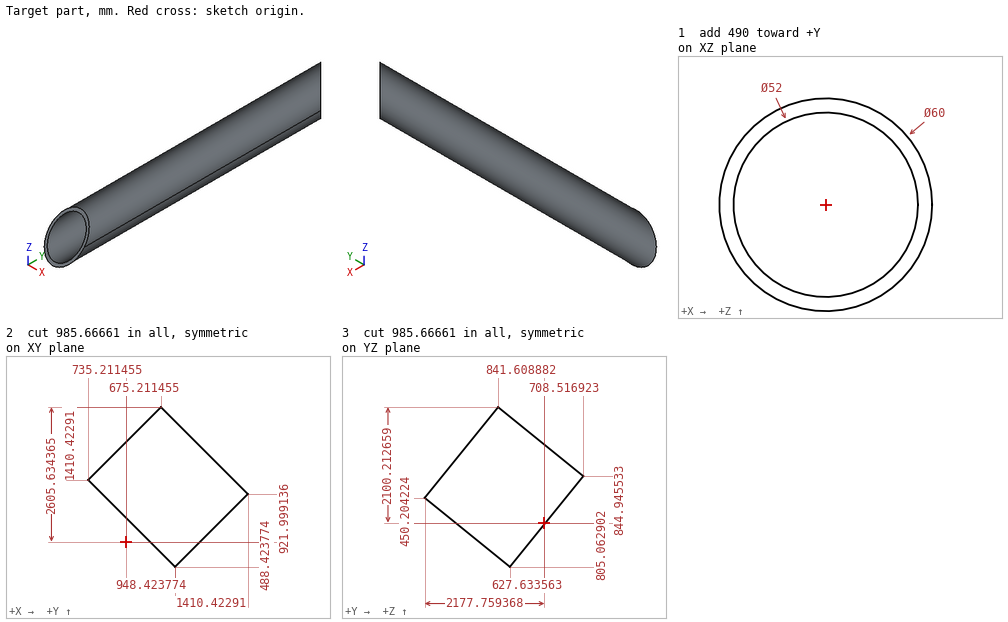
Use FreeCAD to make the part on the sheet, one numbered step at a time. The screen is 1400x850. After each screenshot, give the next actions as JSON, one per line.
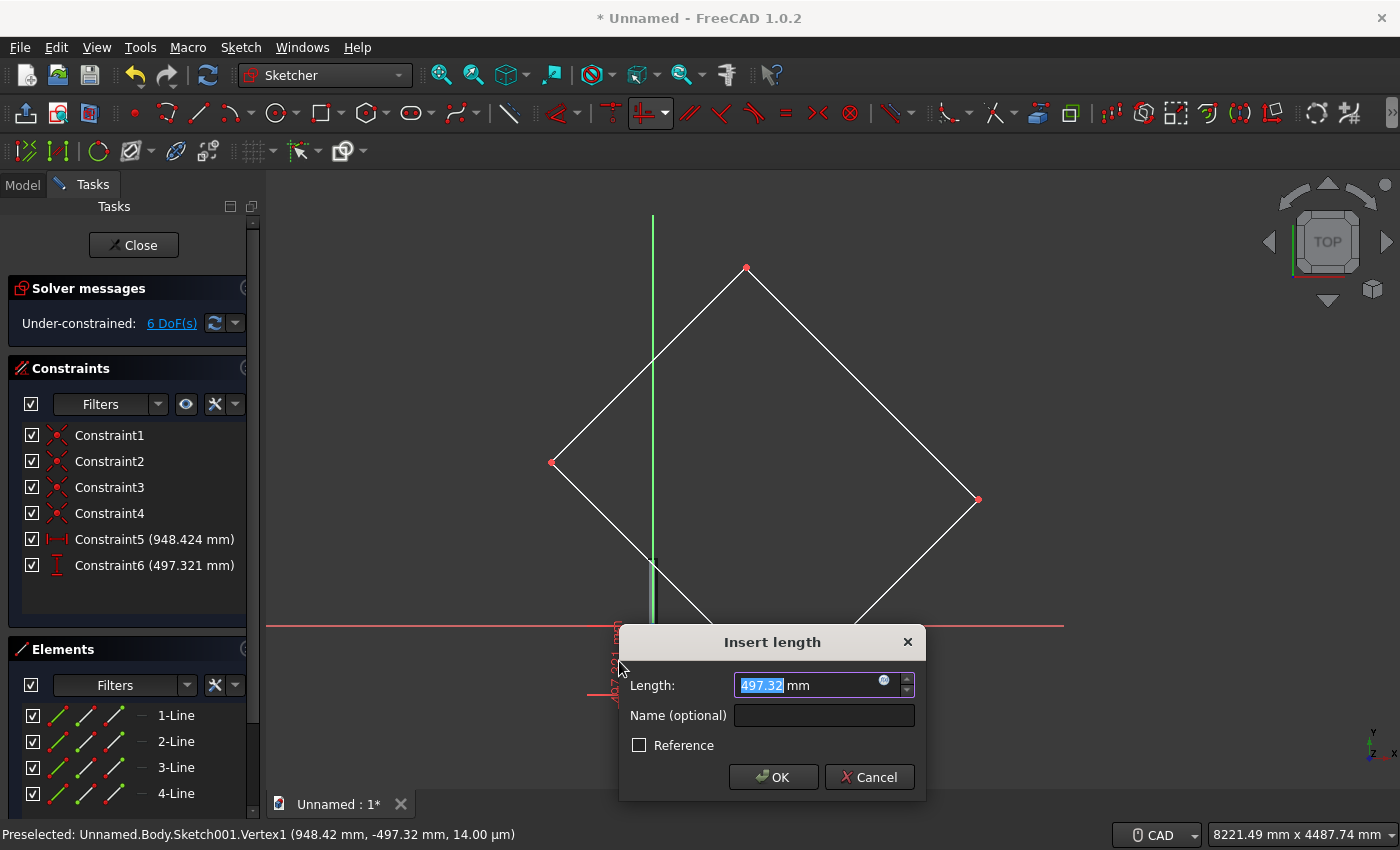
{"action": "type", "text": "488.423774"}
{"action": "key", "text": "Return"}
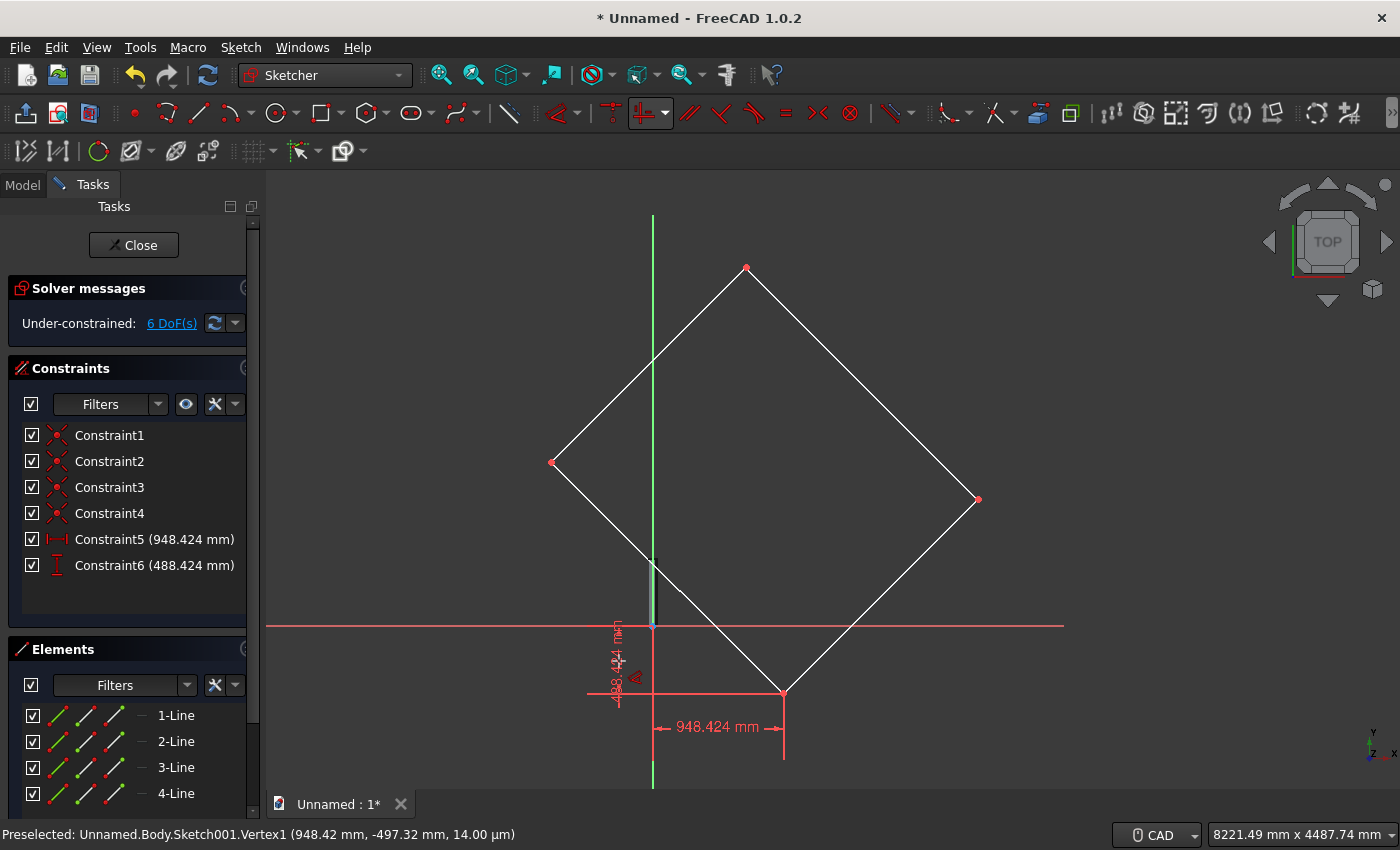
{"action": "left_click", "coordinate": [978, 500]}
{"action": "left_click", "coordinate": [1012, 563]}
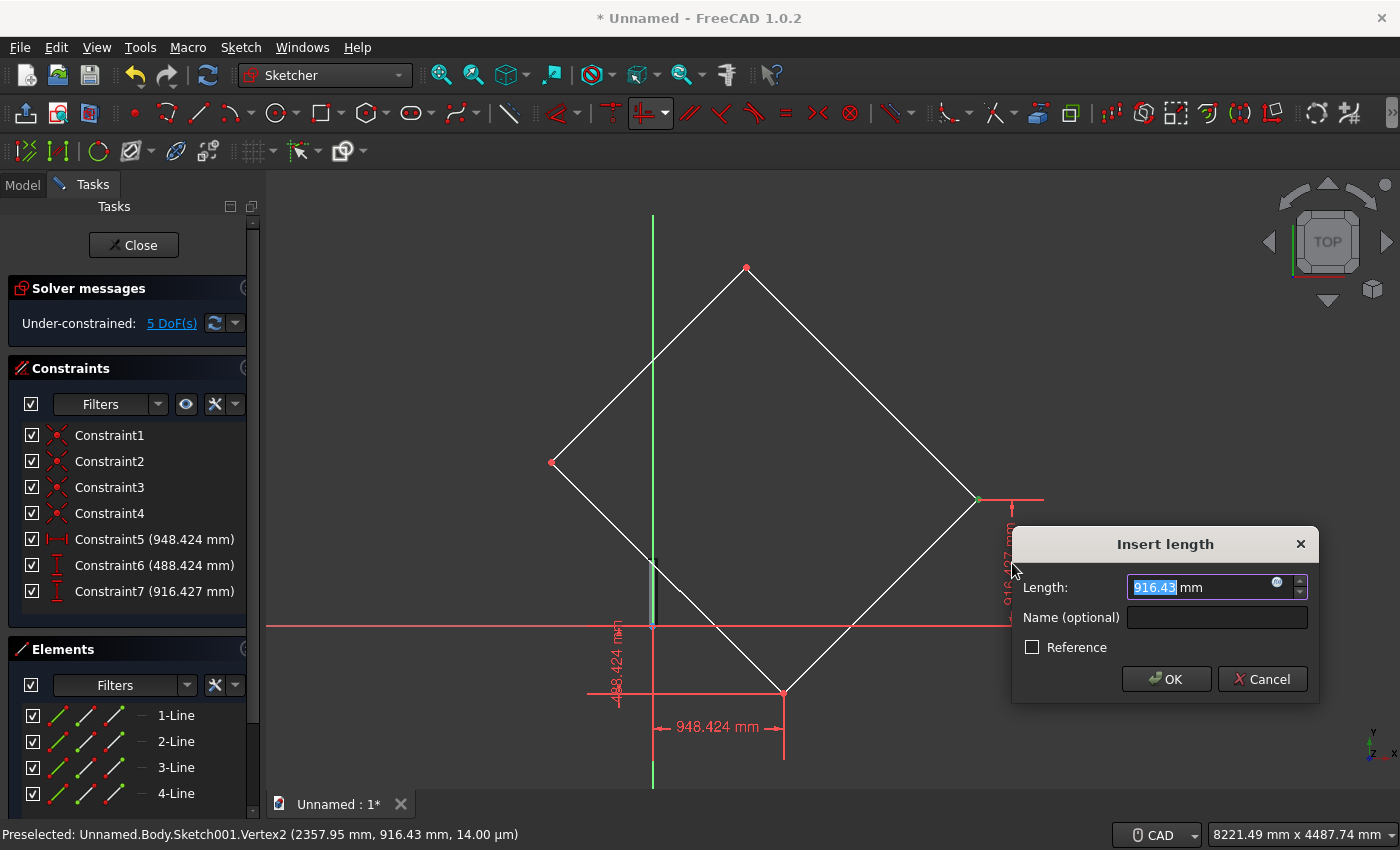
{"action": "type", "text": "921.999136"}
{"action": "key", "text": "Return"}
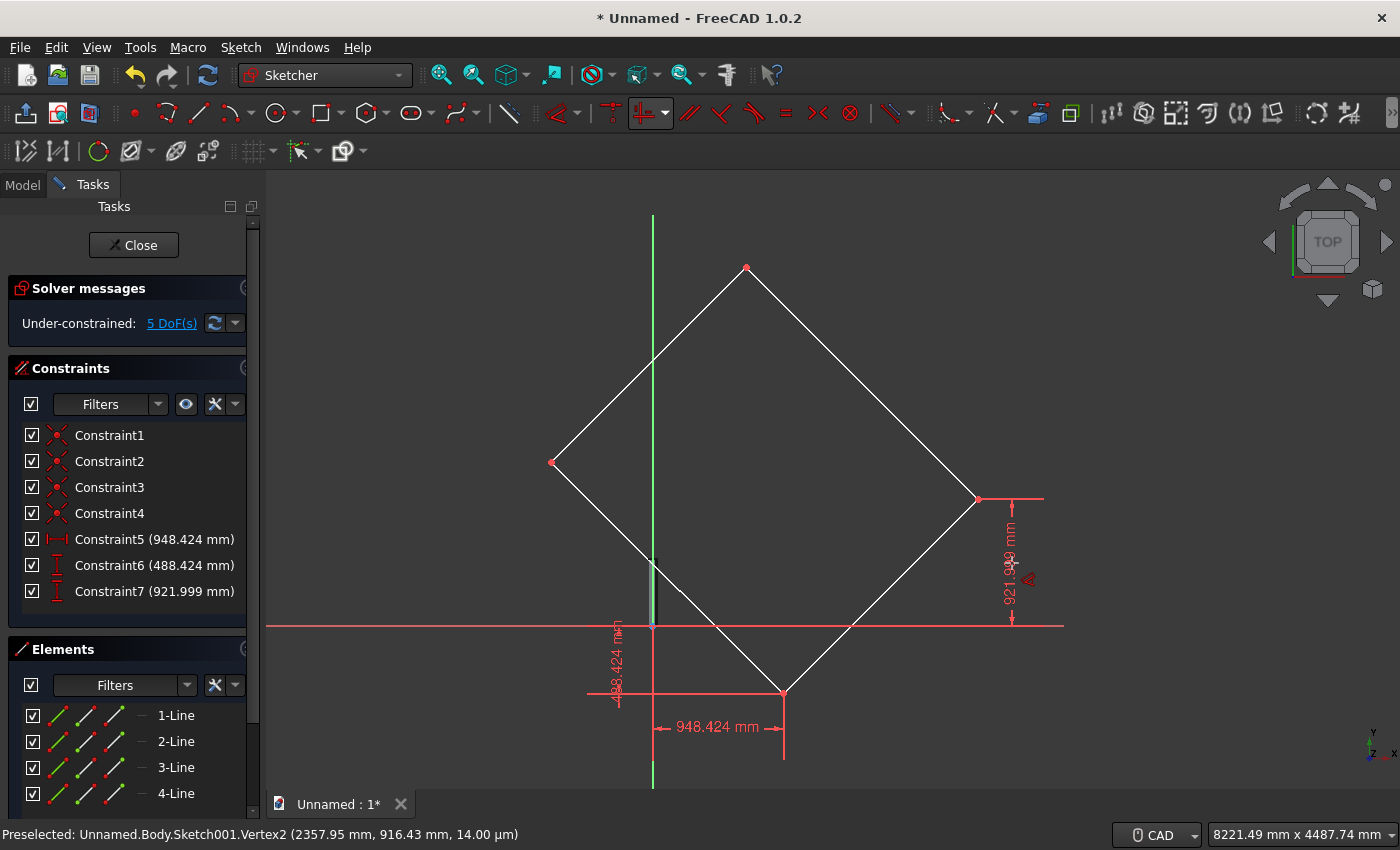
{"action": "left_click", "coordinate": [746, 268]}
{"action": "left_click", "coordinate": [699, 234]}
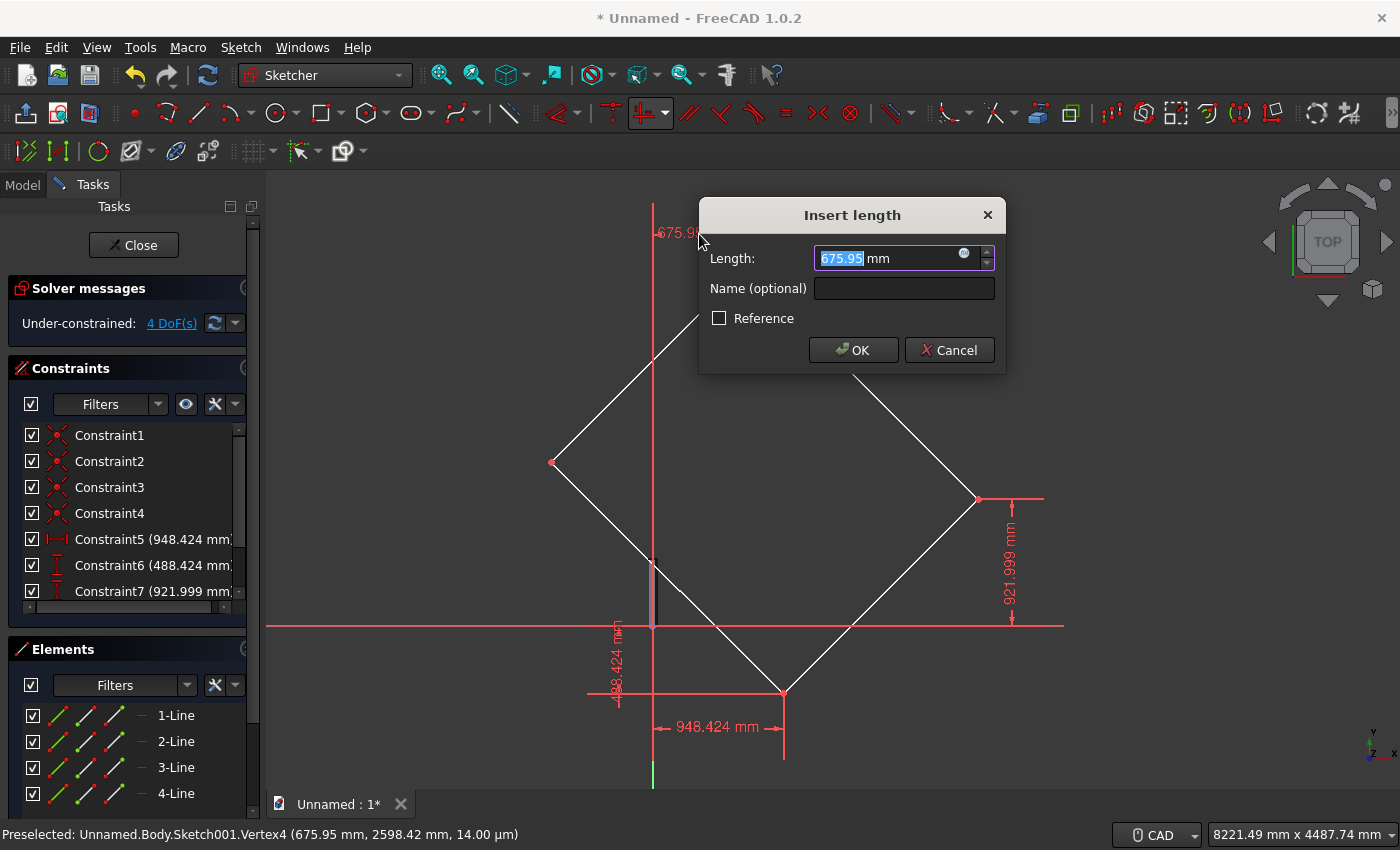
{"action": "type", "text": "675.211455"}
{"action": "key", "text": "Return"}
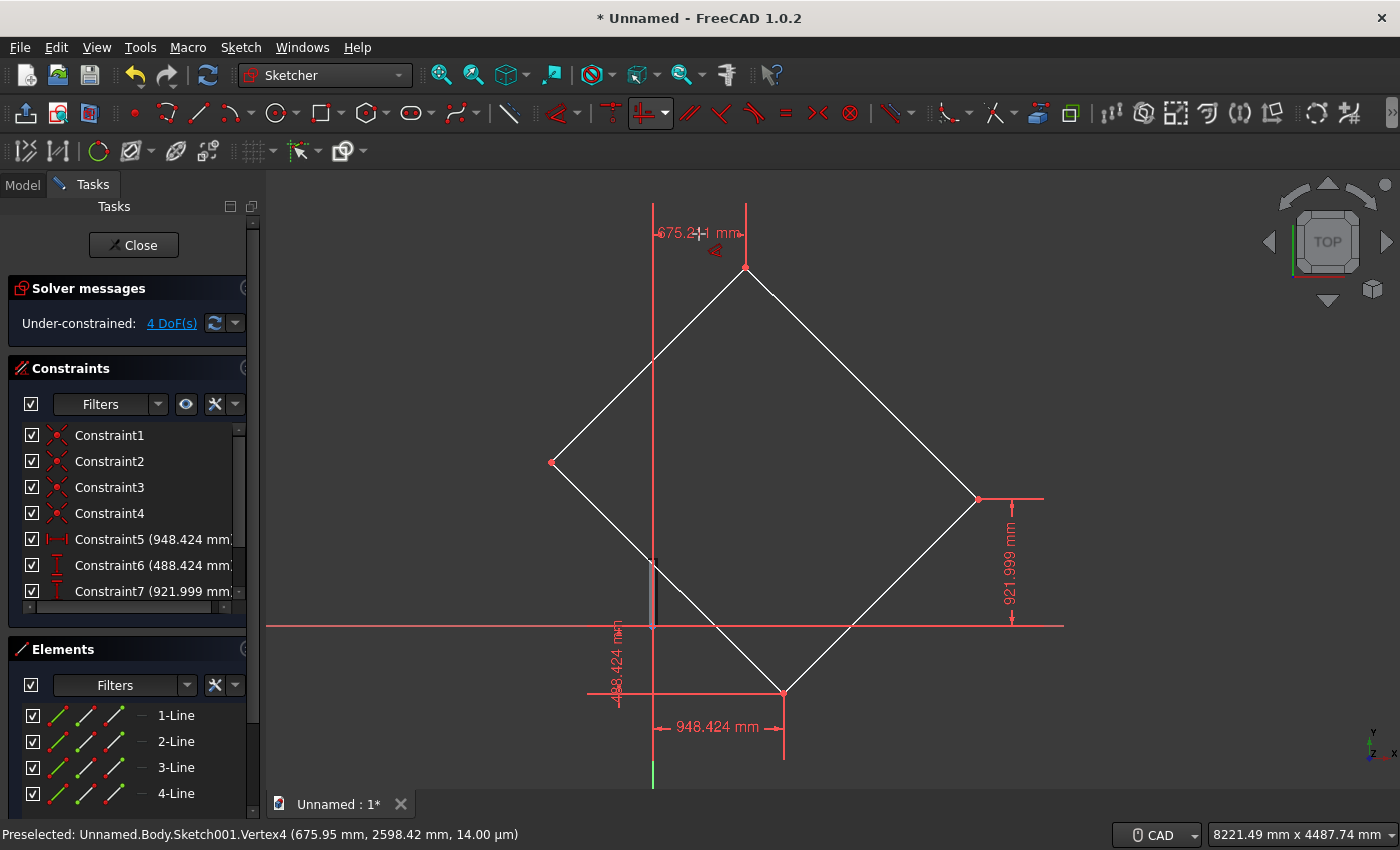
{"action": "left_click", "coordinate": [551, 463]}
{"action": "left_click", "coordinate": [625, 429]}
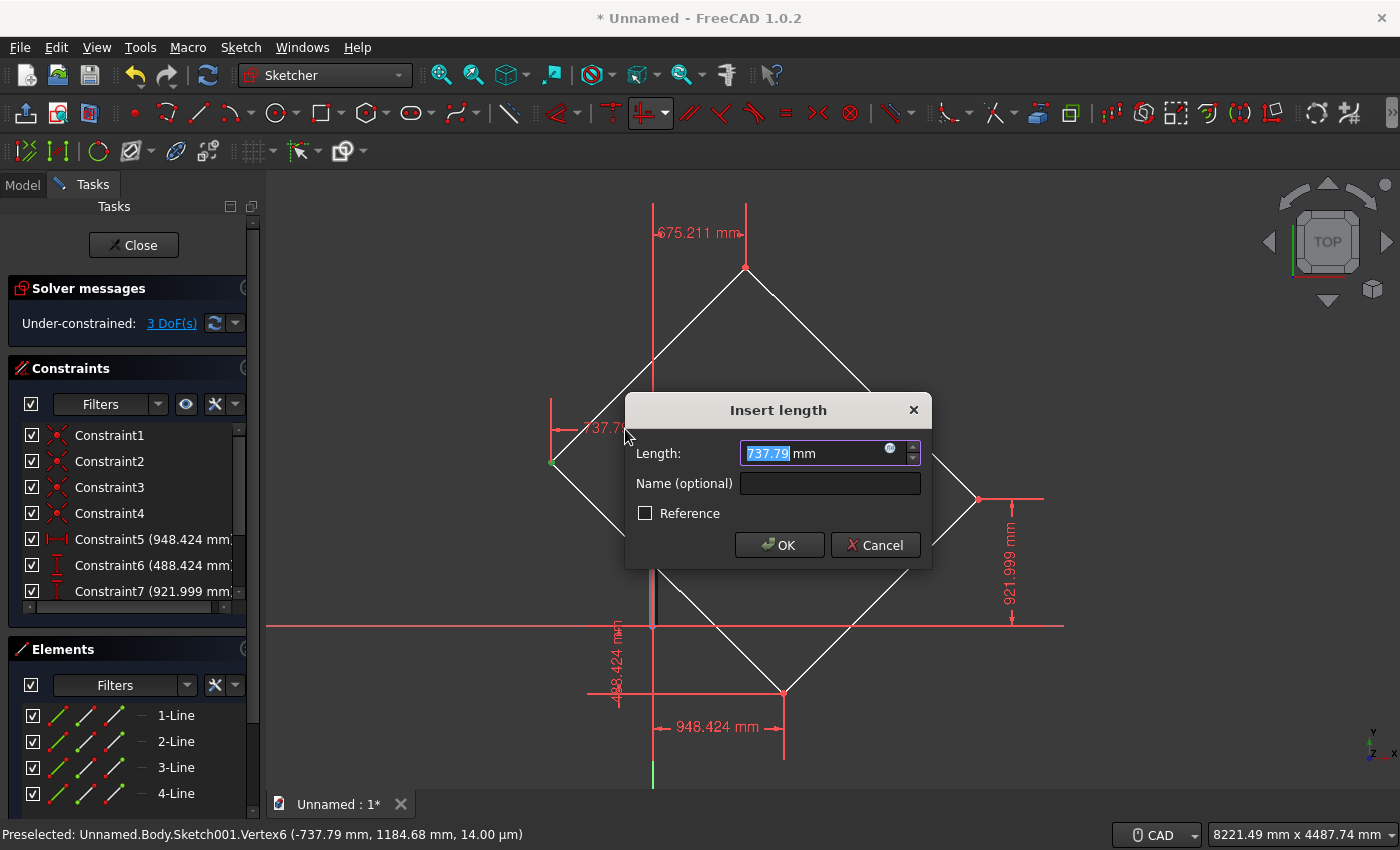
{"action": "type", "text": "735.211455"}
{"action": "key", "text": "Return"}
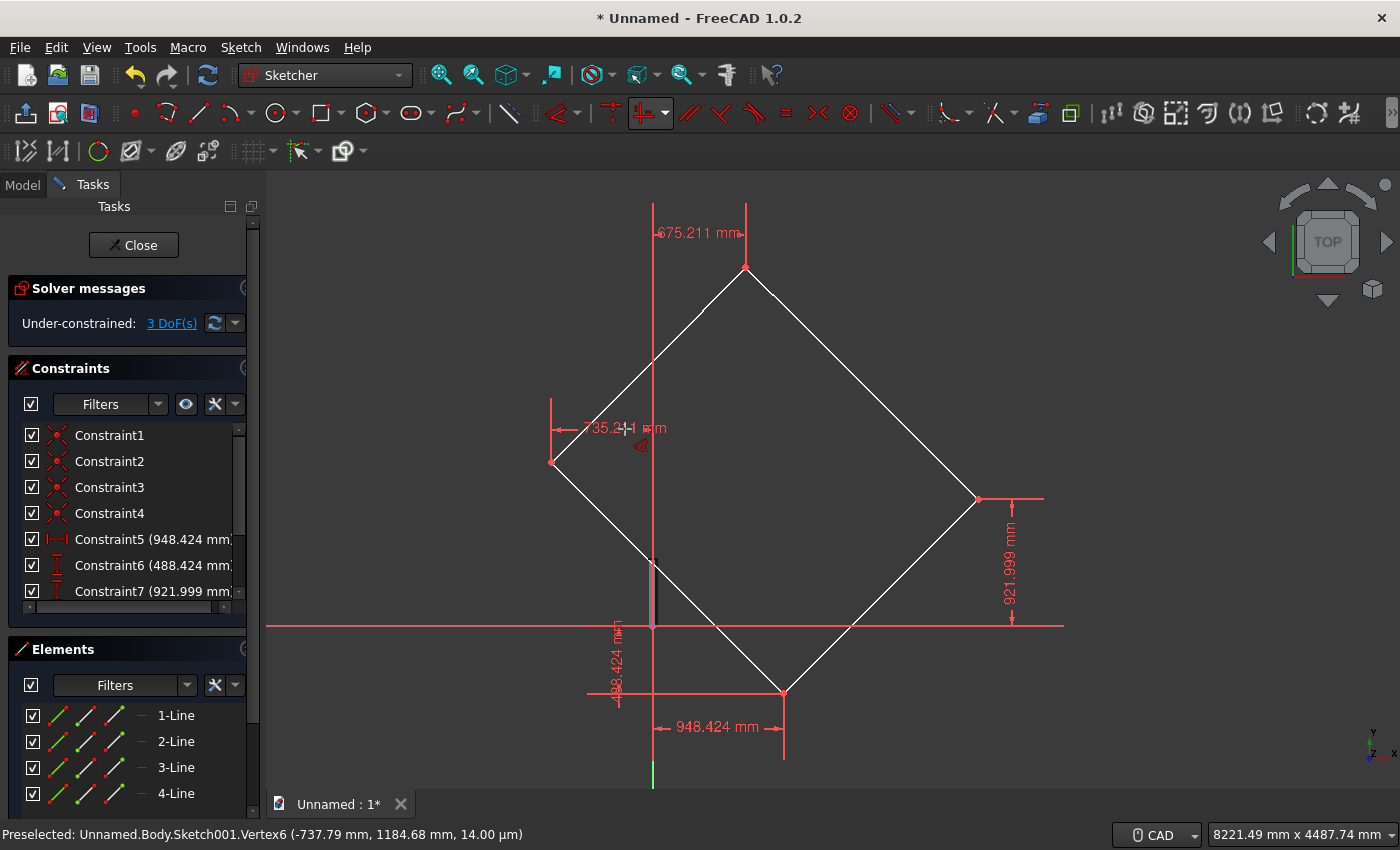
{"action": "scroll", "coordinate": [842, 635], "scroll_direction": "up", "scroll_amount": 3}